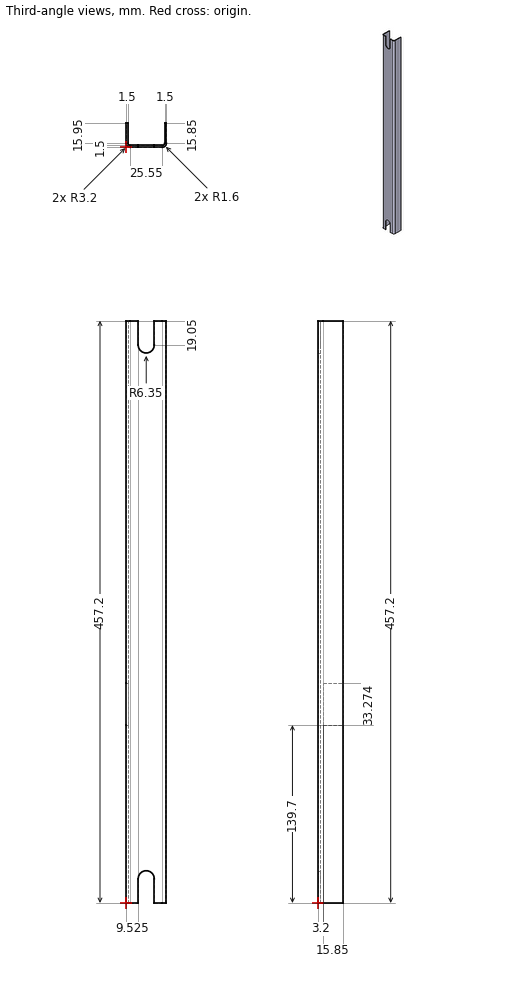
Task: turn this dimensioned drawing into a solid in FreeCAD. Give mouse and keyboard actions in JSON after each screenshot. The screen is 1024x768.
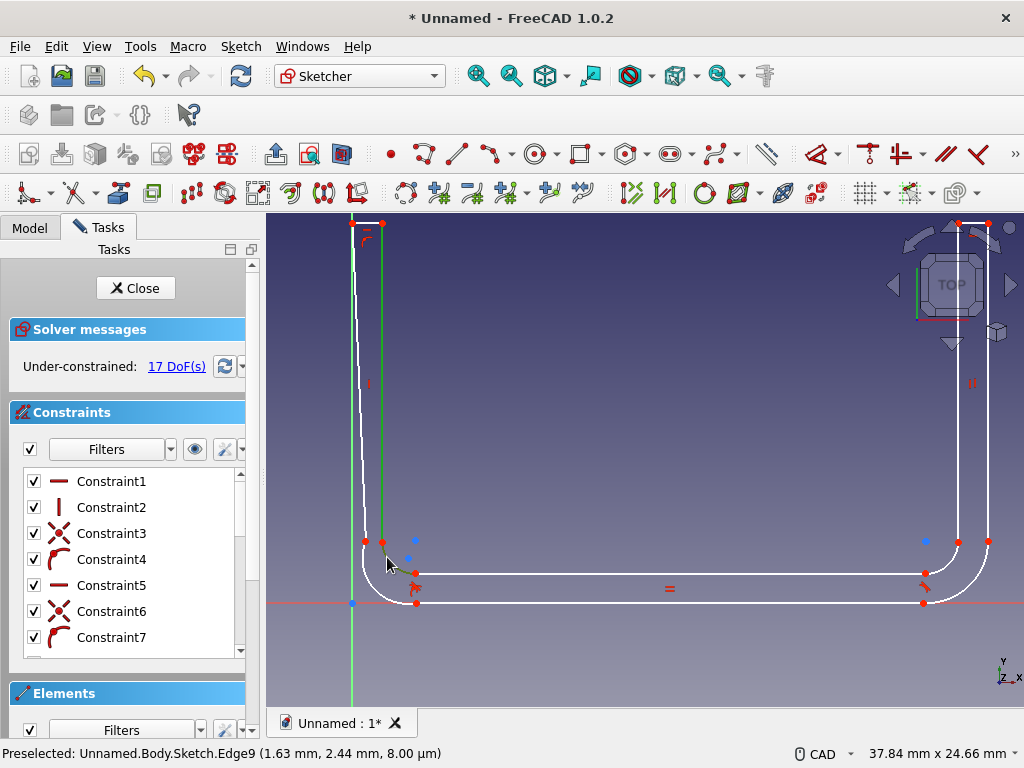
{"action": "key", "text": "t"}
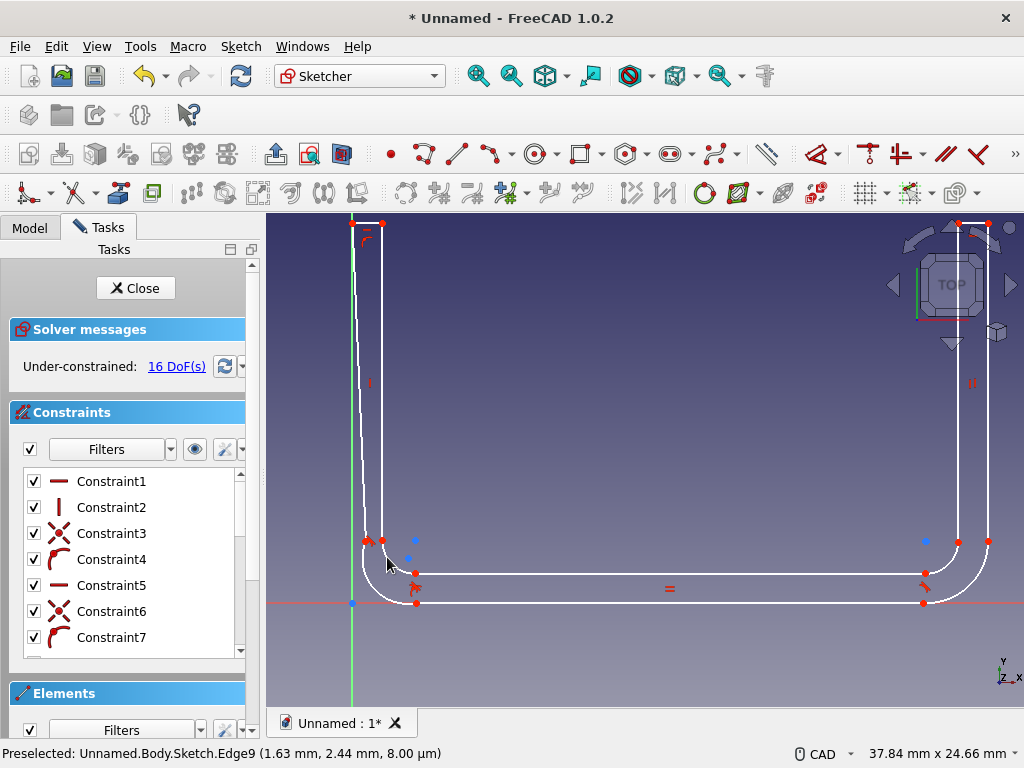
{"action": "scroll", "coordinate": [362, 446], "scroll_direction": "up", "scroll_amount": 2}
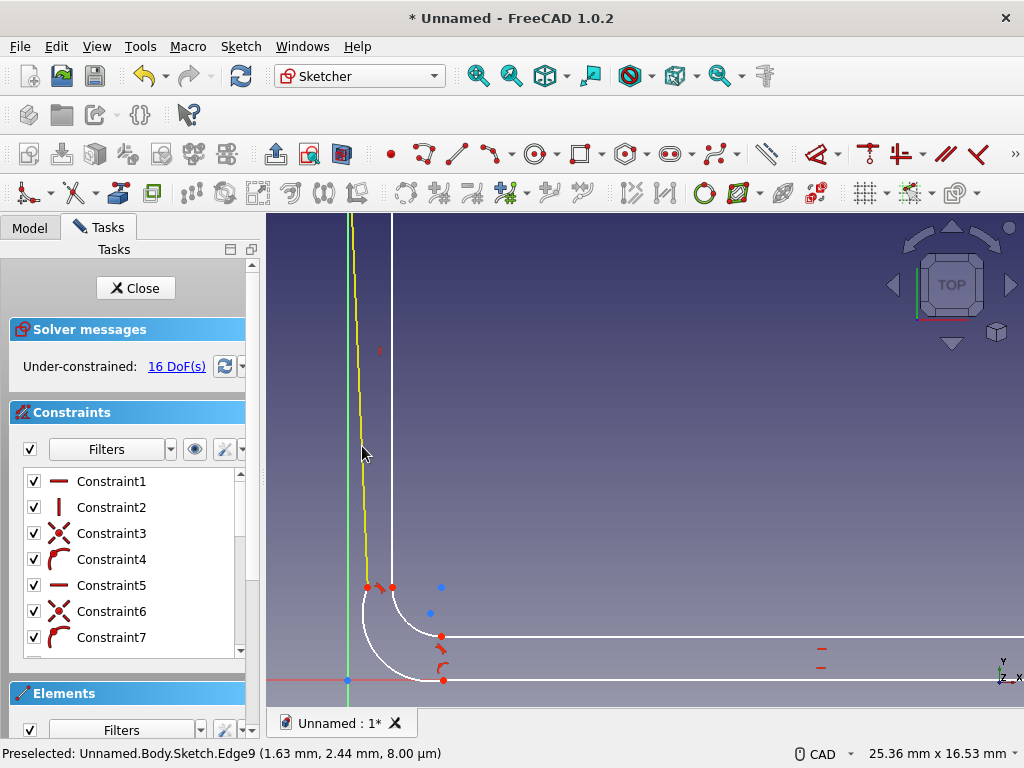
{"action": "left_click", "coordinate": [362, 445]}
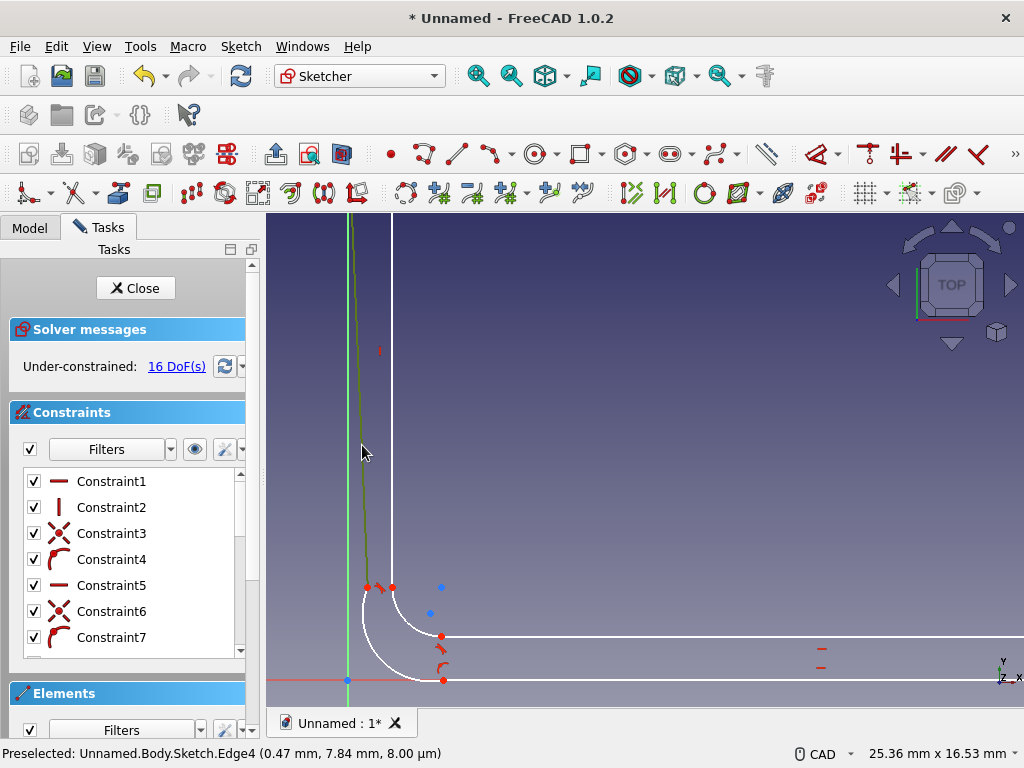
{"action": "left_click", "coordinate": [365, 631]}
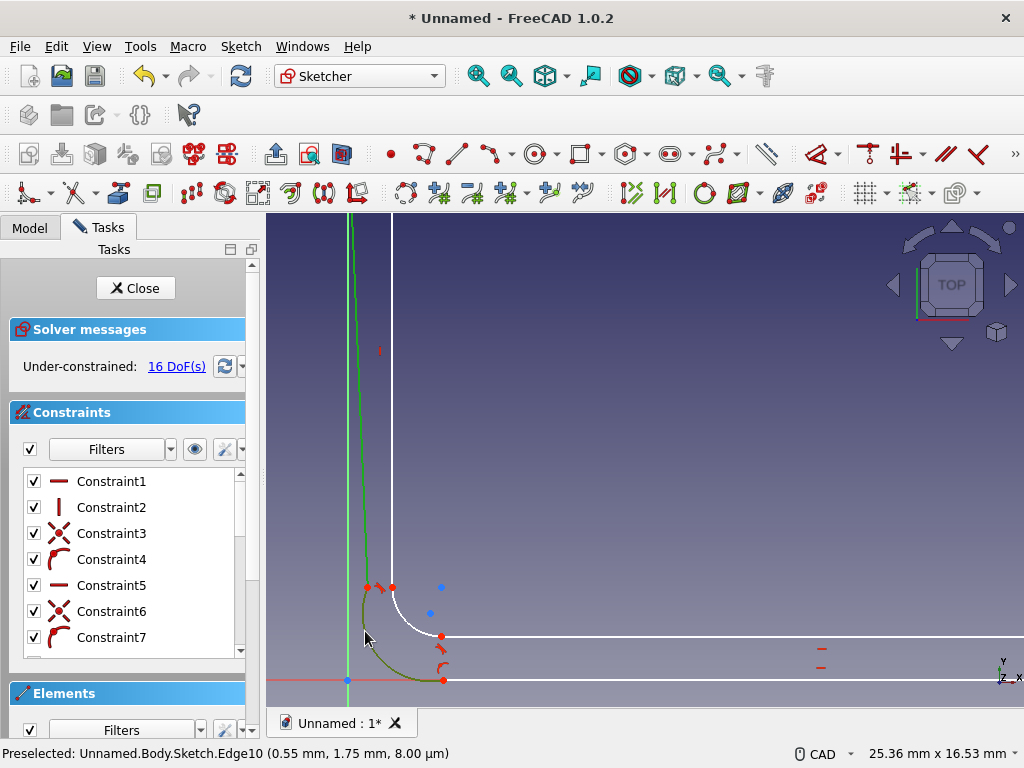
{"action": "key", "text": "t"}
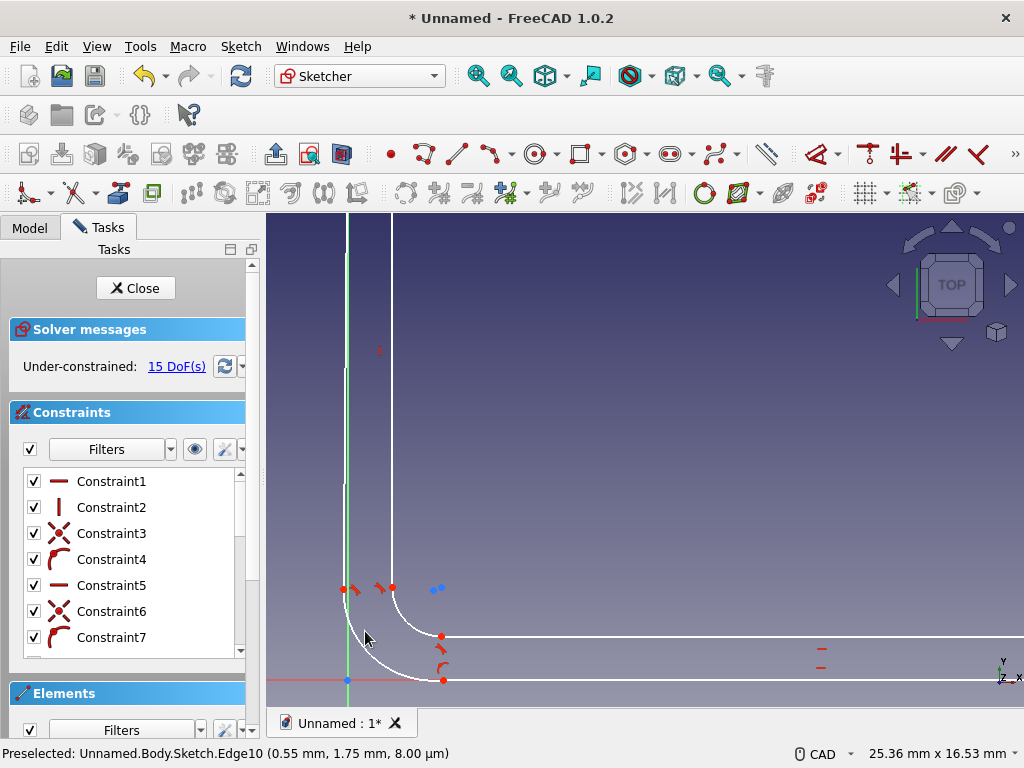
{"action": "scroll", "coordinate": [376, 513], "scroll_direction": "down", "scroll_amount": 4}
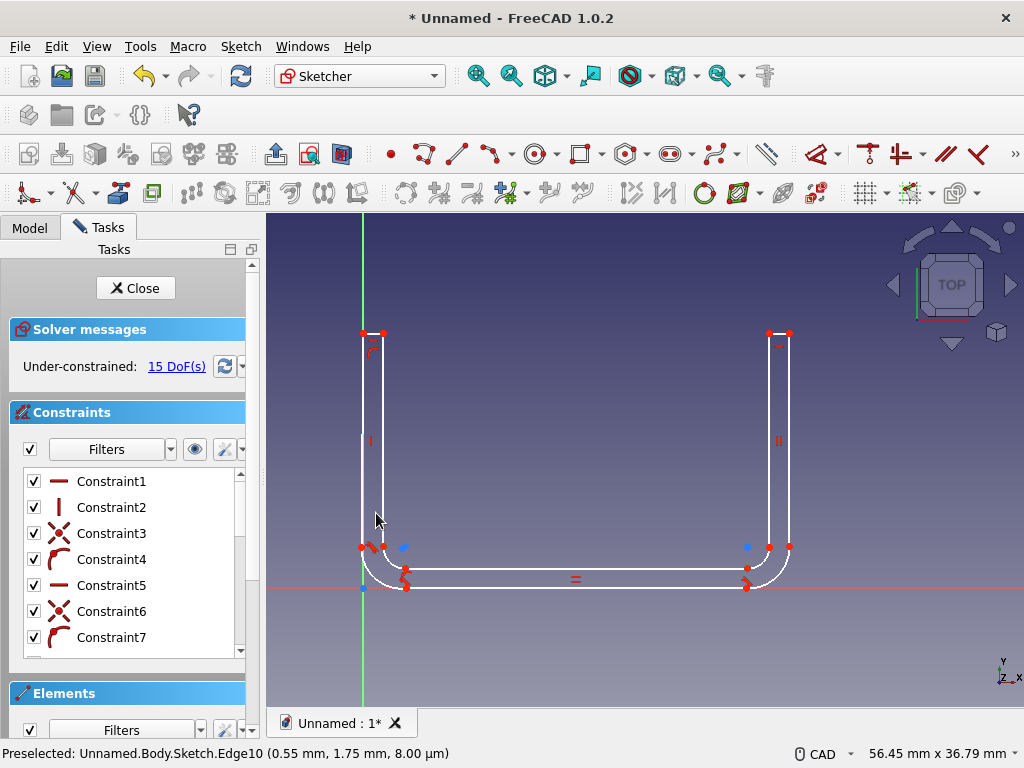
{"action": "left_click", "coordinate": [508, 588]}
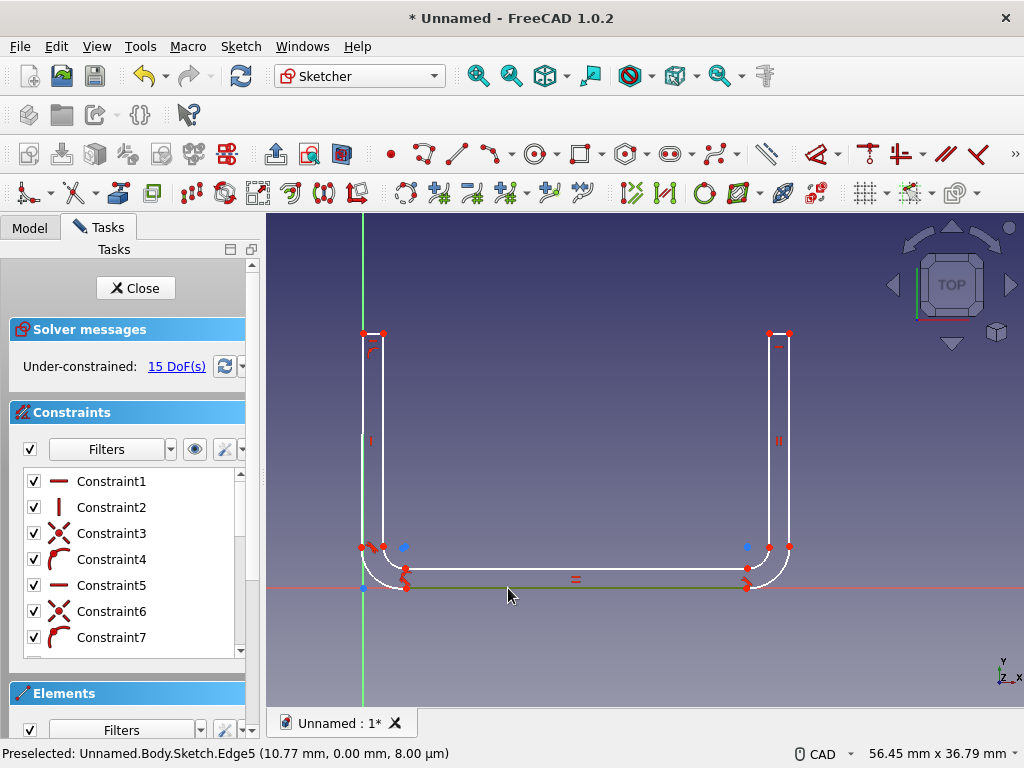
{"action": "left_click", "coordinate": [366, 568]}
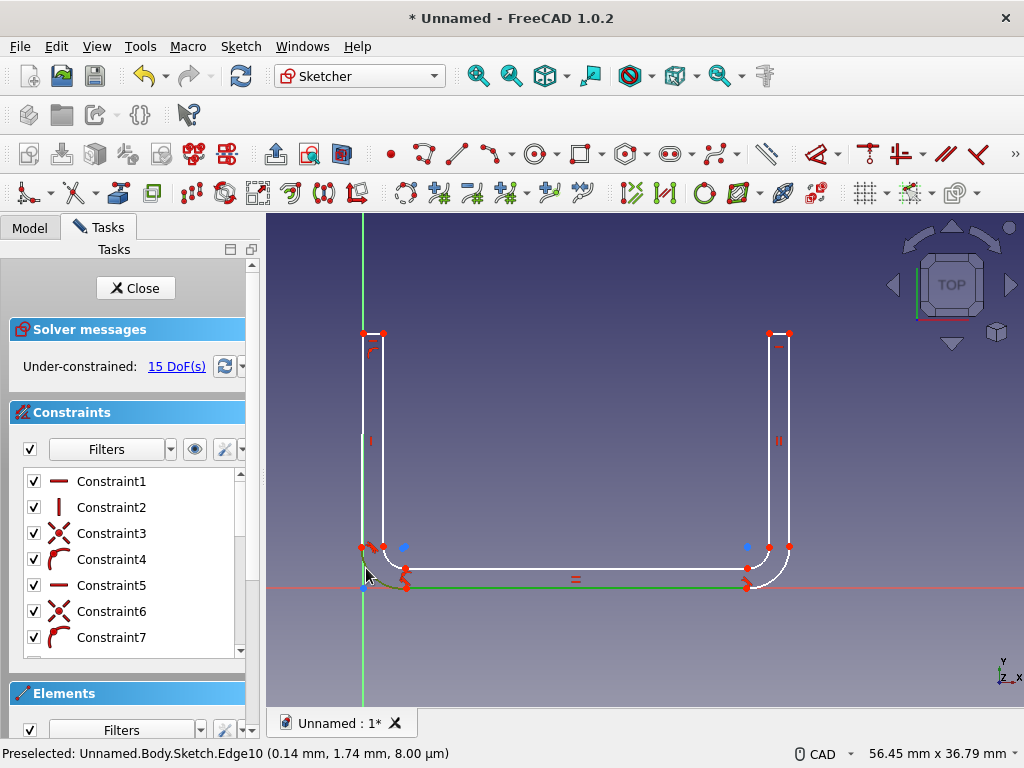
{"action": "key", "text": "t"}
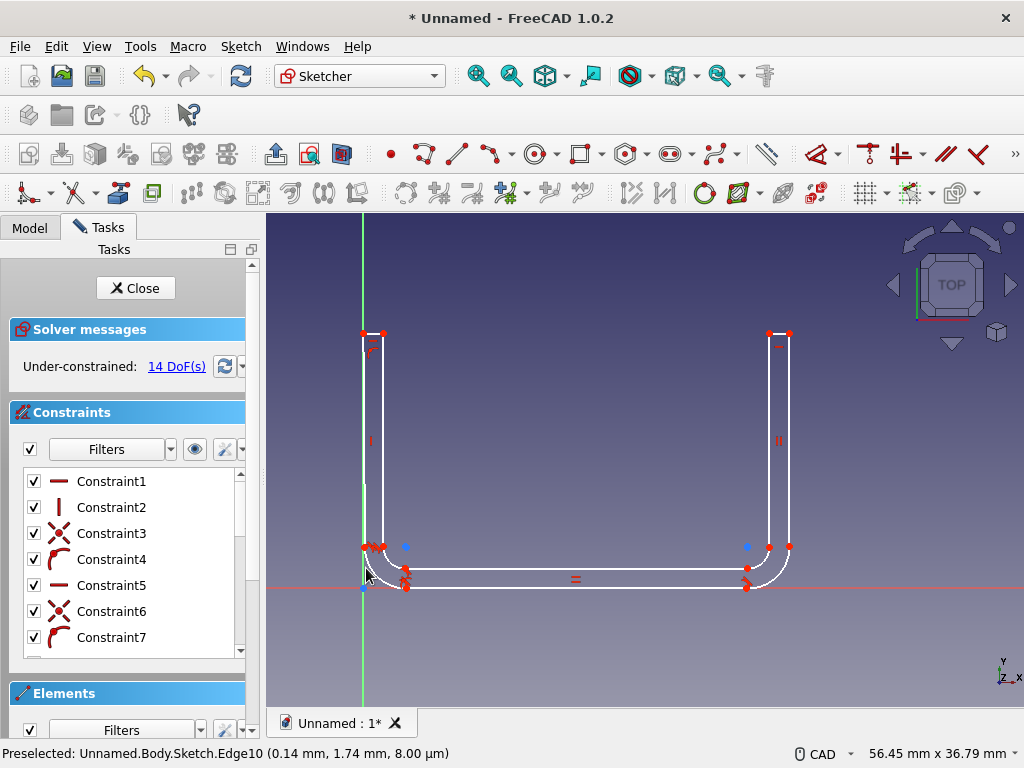
{"action": "left_click", "coordinate": [508, 588]}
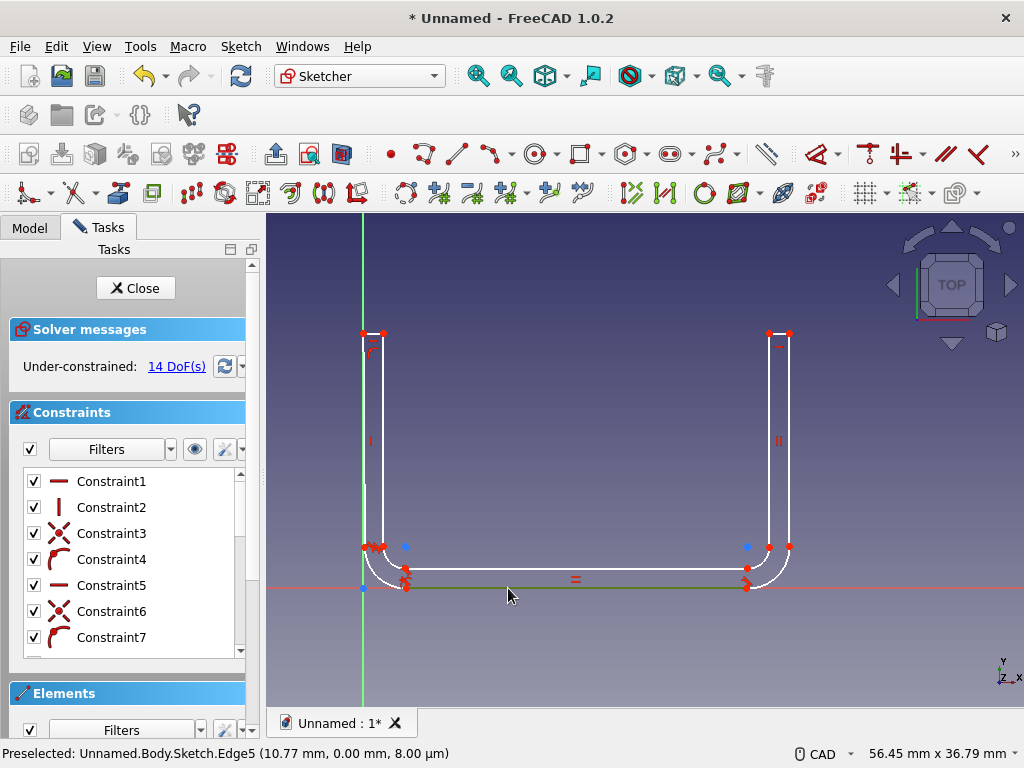
{"action": "left_click", "coordinate": [785, 566]}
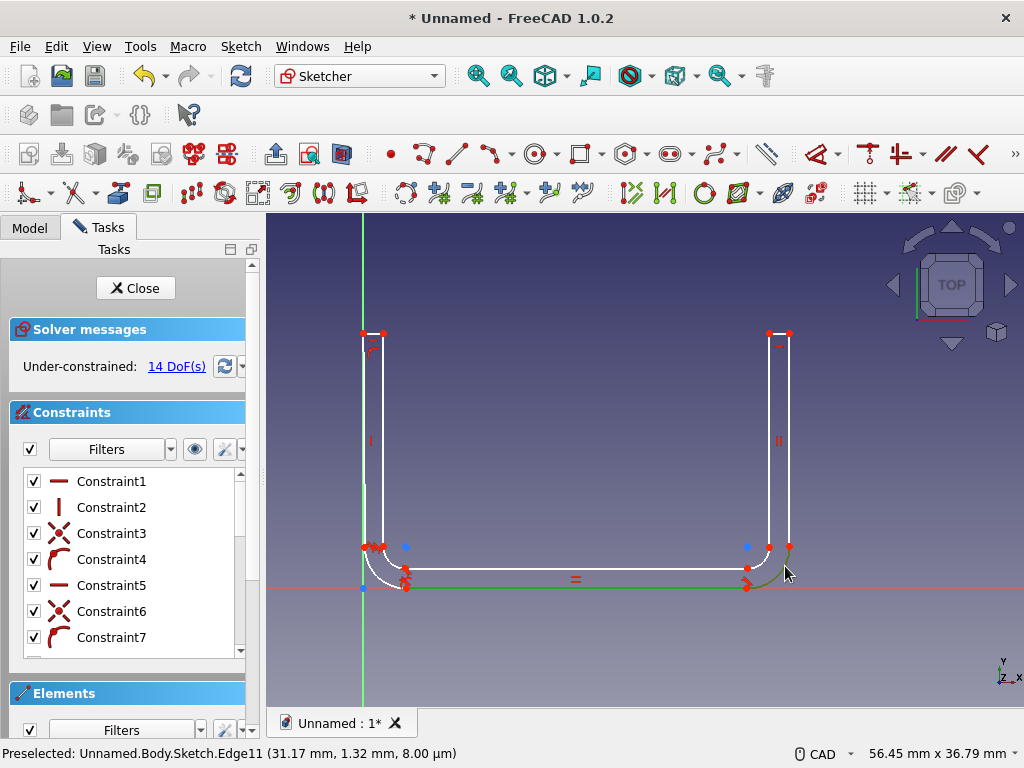
{"action": "key", "text": "t"}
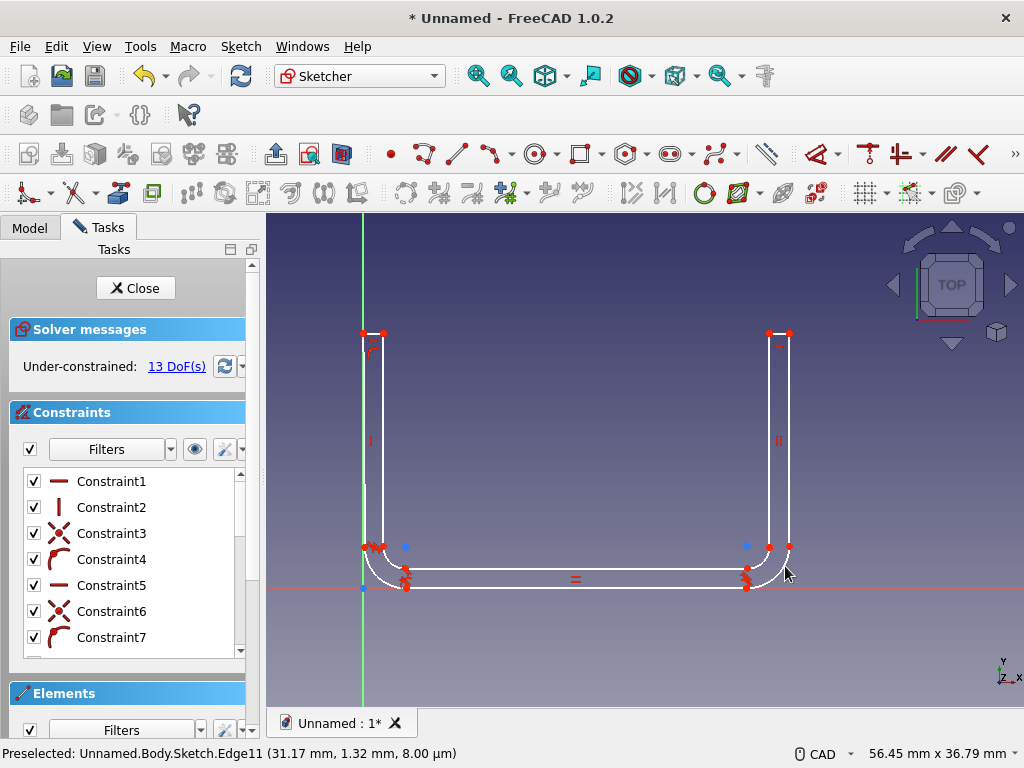
{"action": "left_click", "coordinate": [789, 483]}